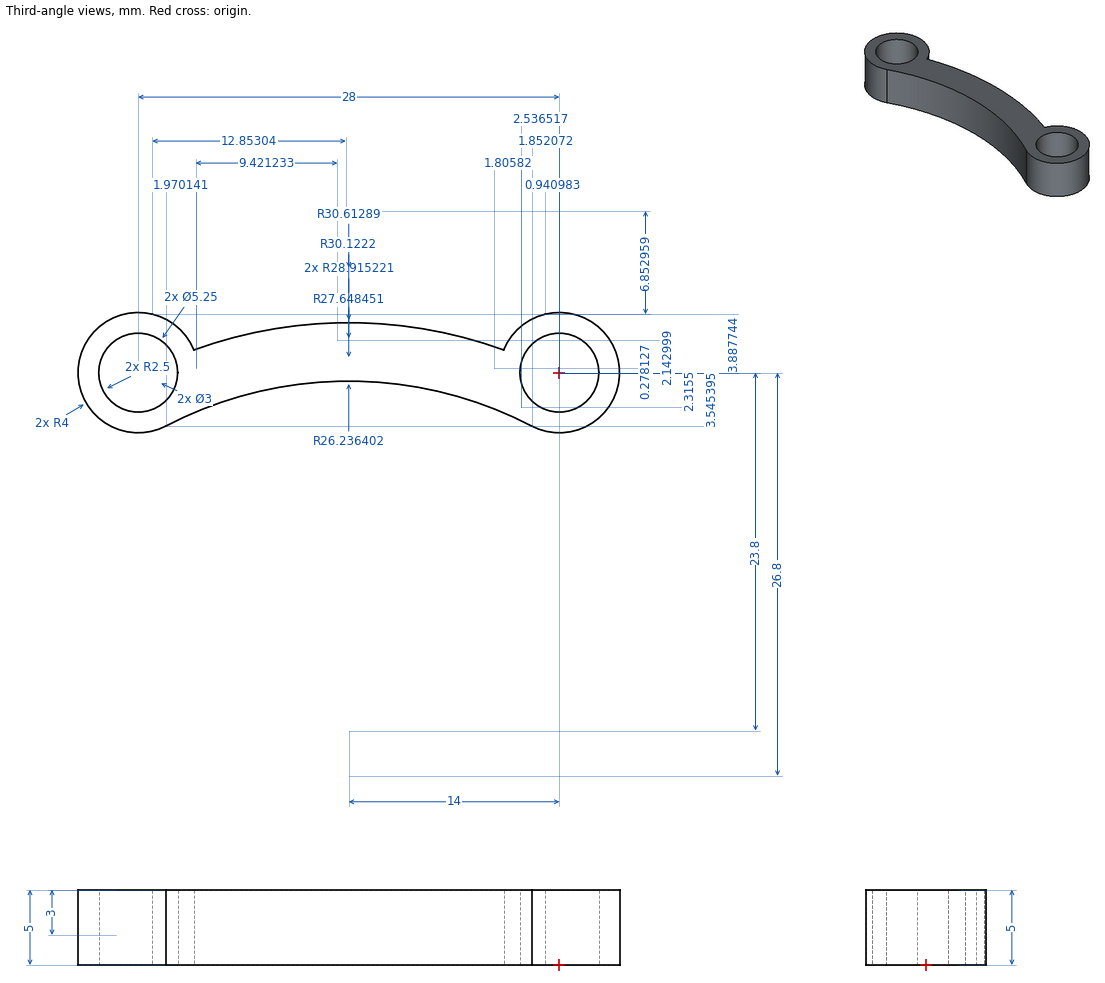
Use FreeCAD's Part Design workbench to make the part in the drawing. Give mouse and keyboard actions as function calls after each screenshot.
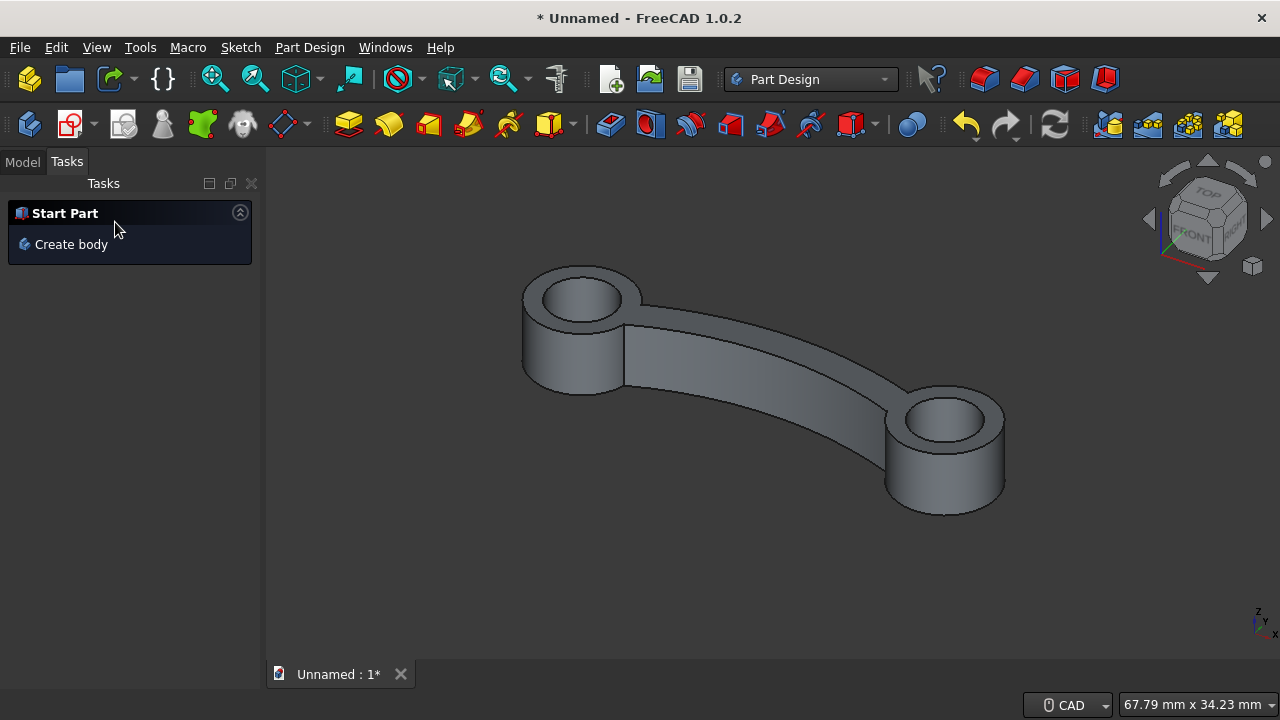
click(897, 403)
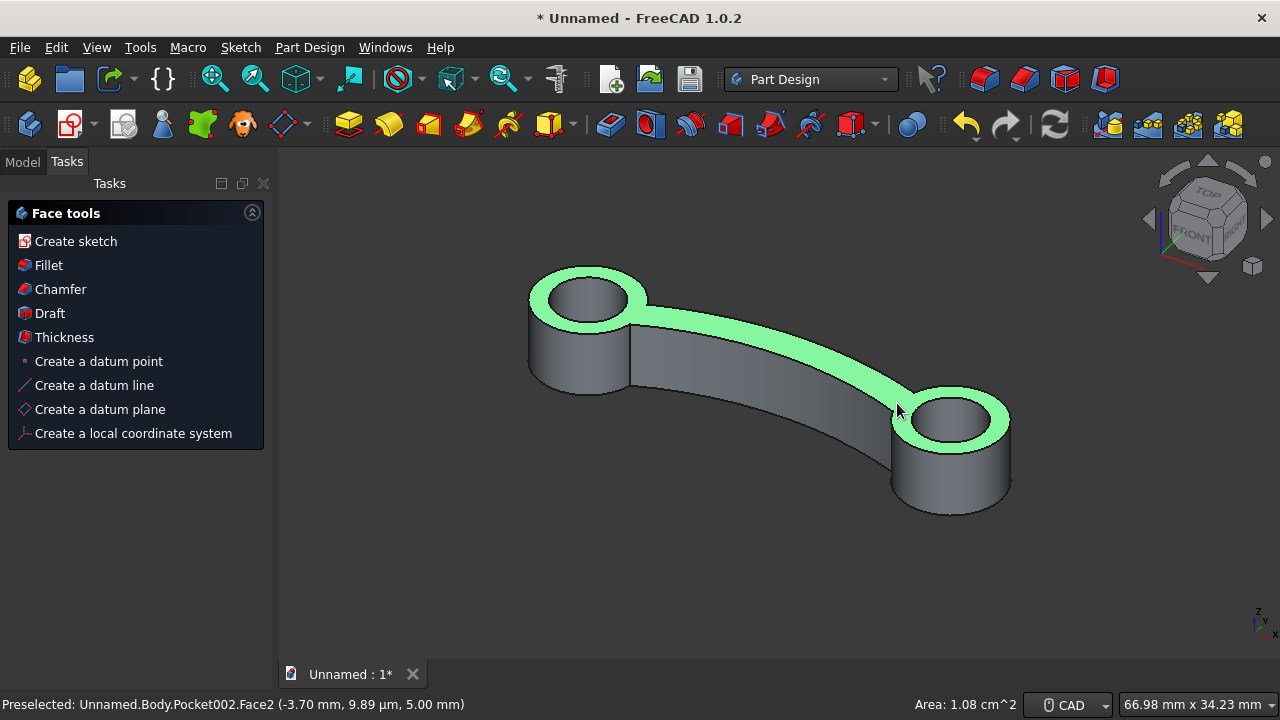
click(70, 124)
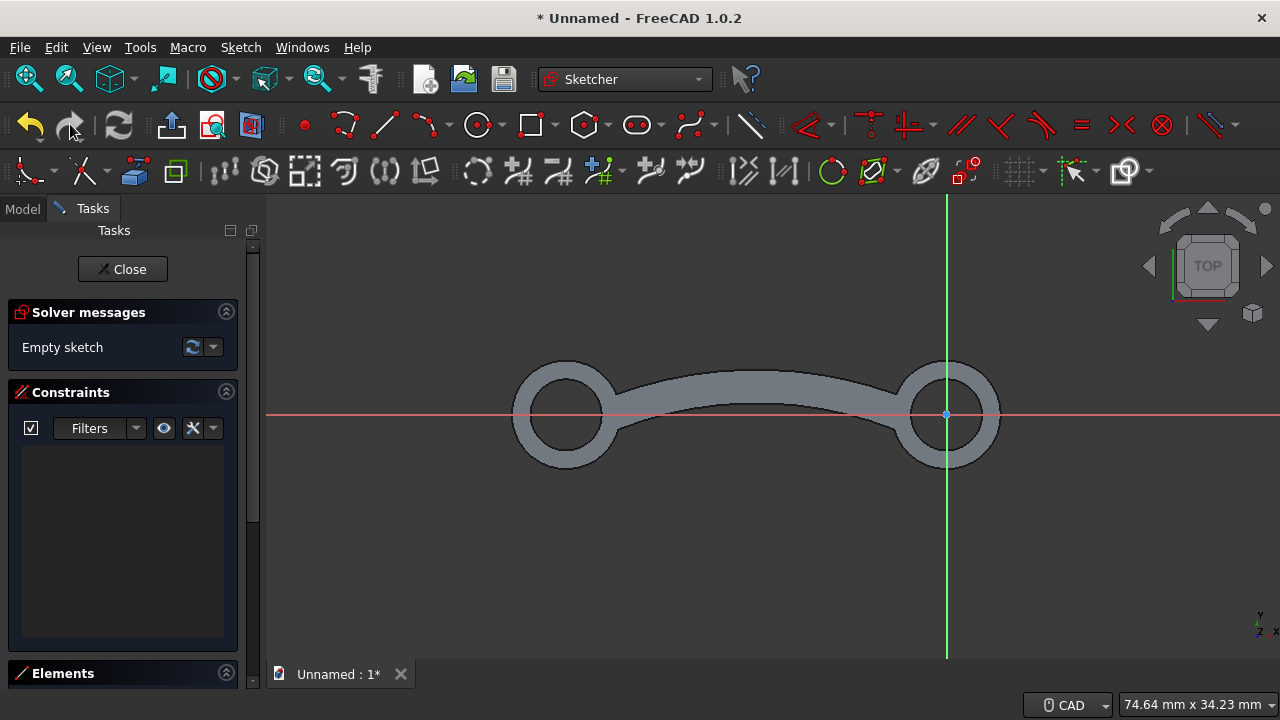
scroll(900, 420, up, 2)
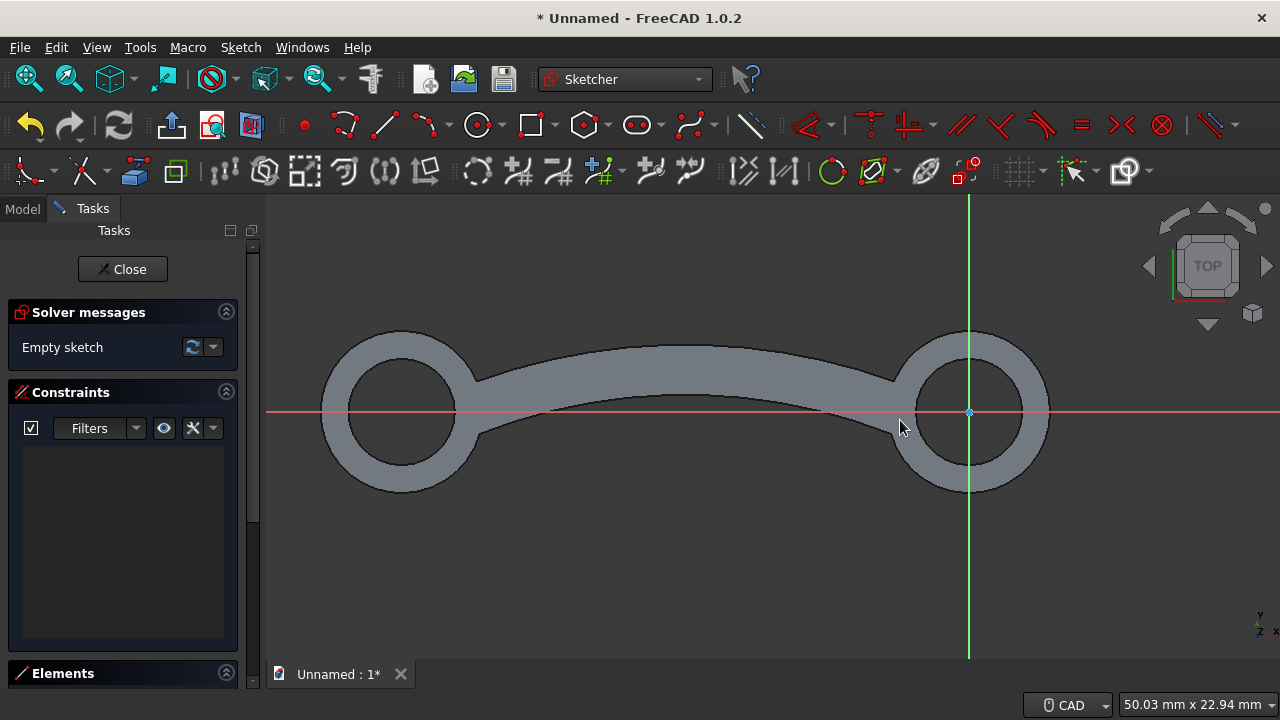
click(346, 126)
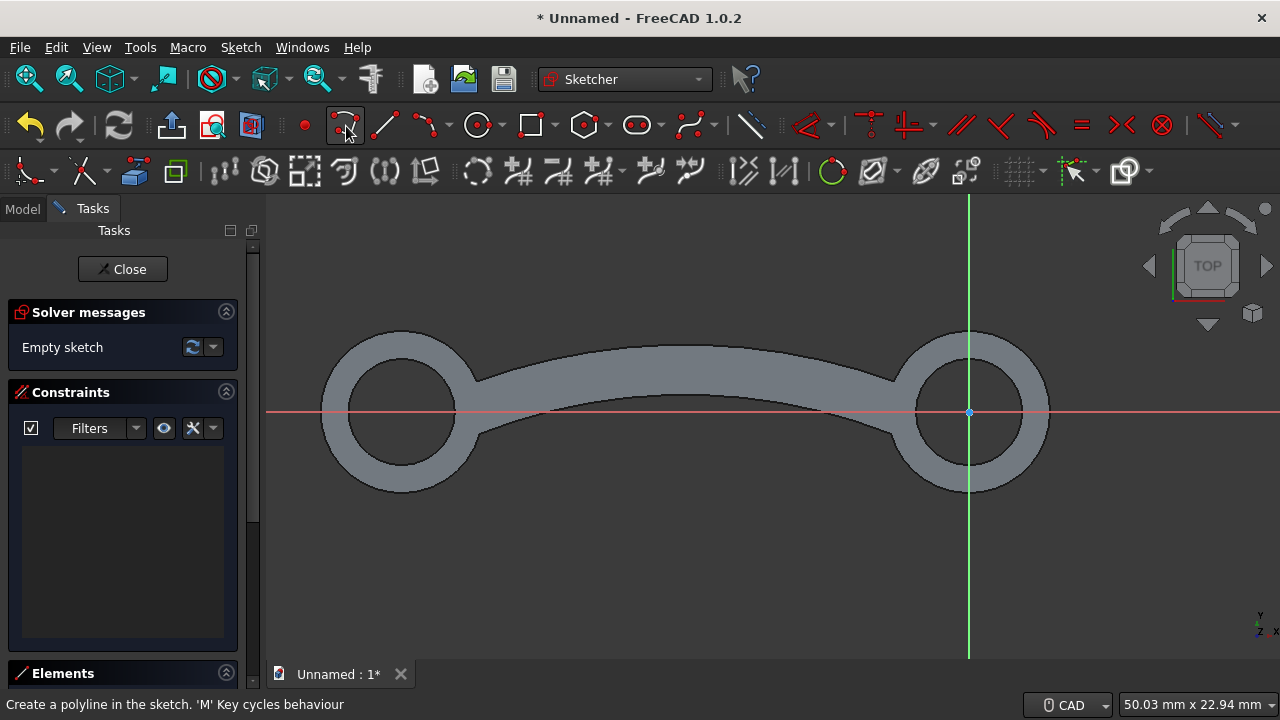
click(932, 484)
click(918, 459)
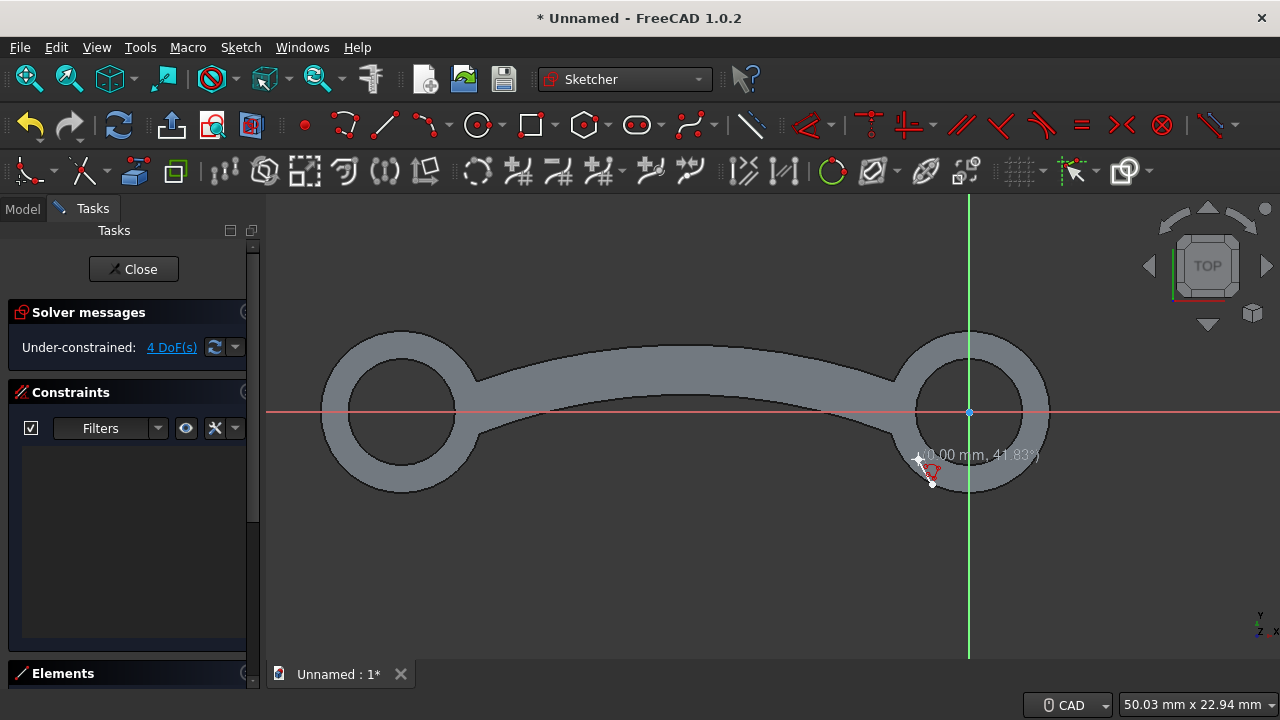
scroll(881, 406, up, 6)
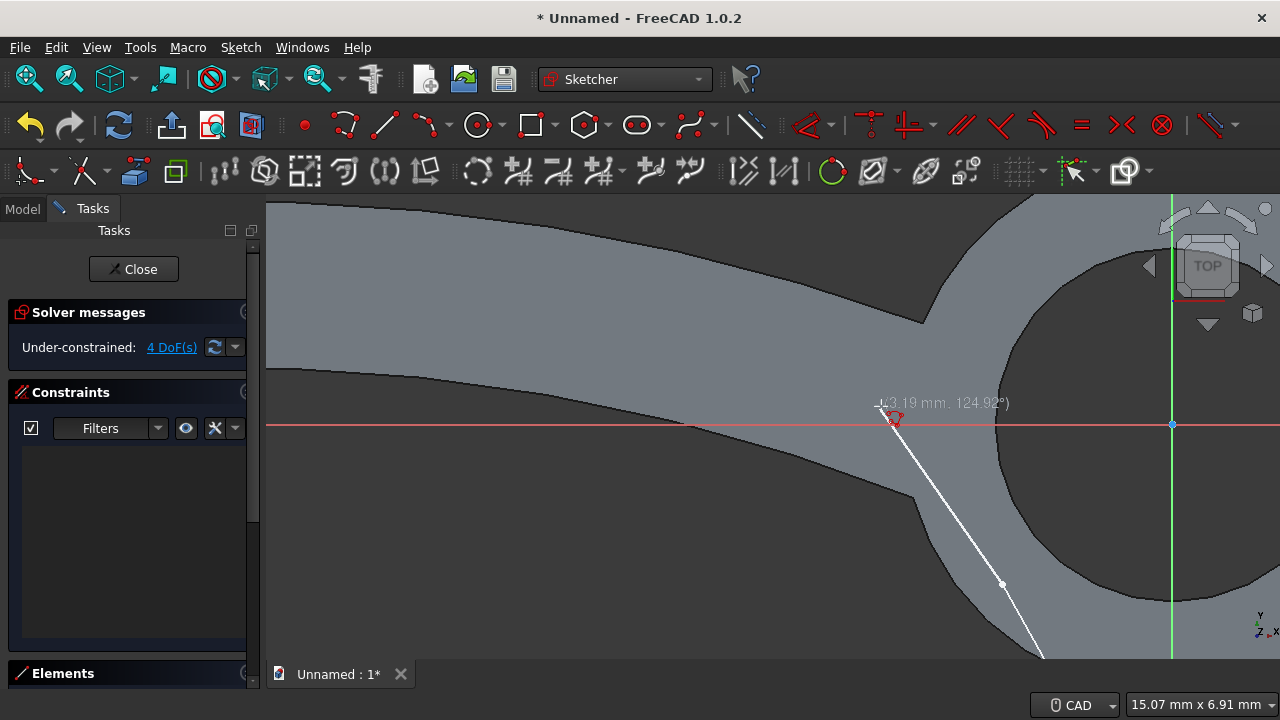
click(880, 406)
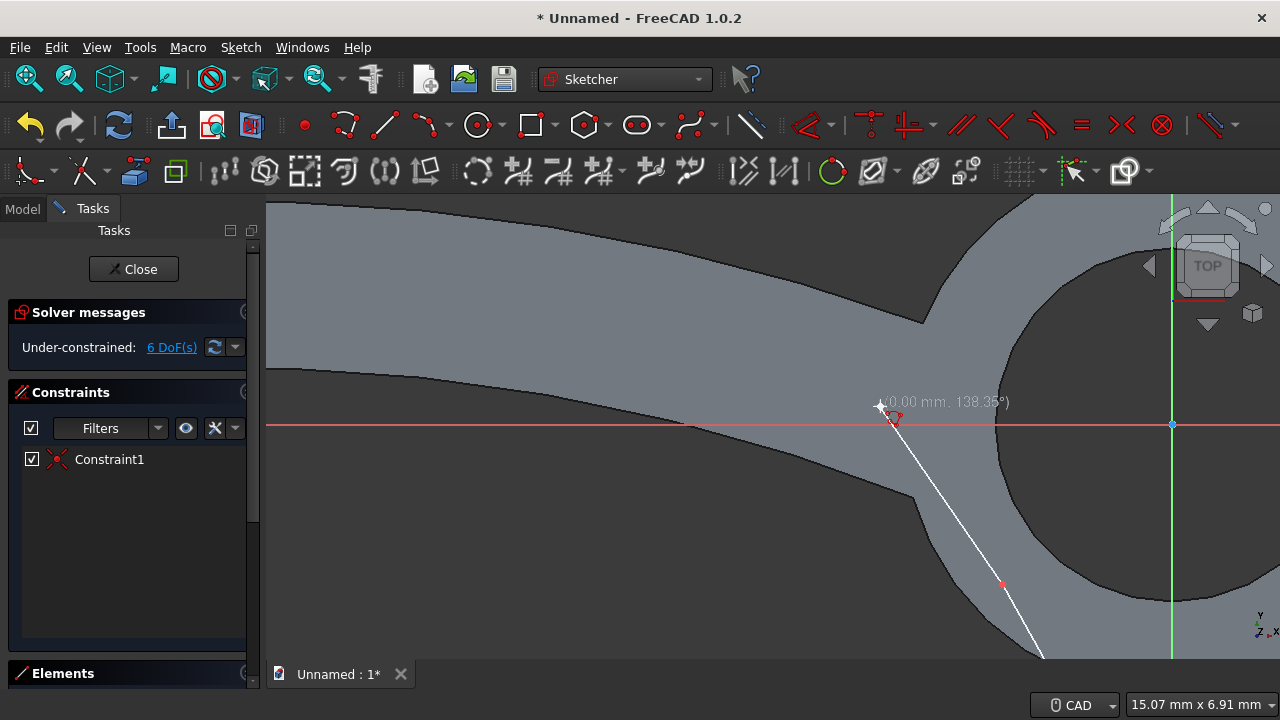
scroll(882, 407, down, 6)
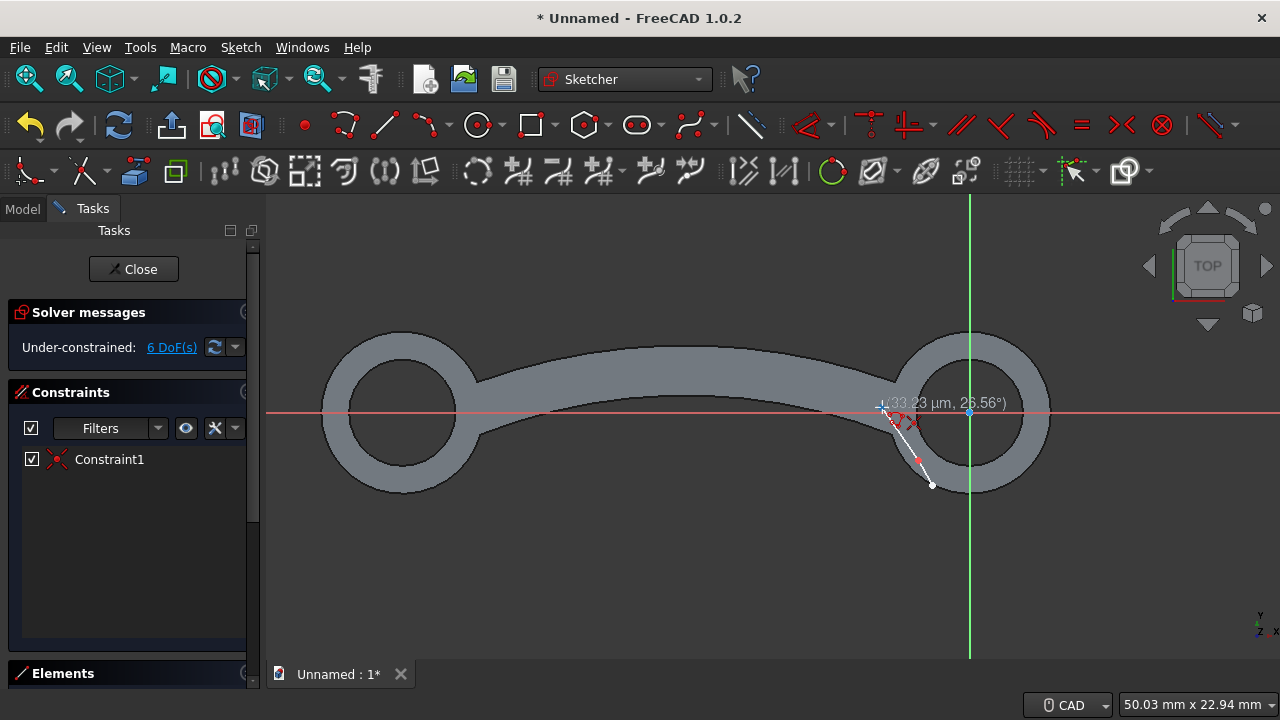
click(671, 369)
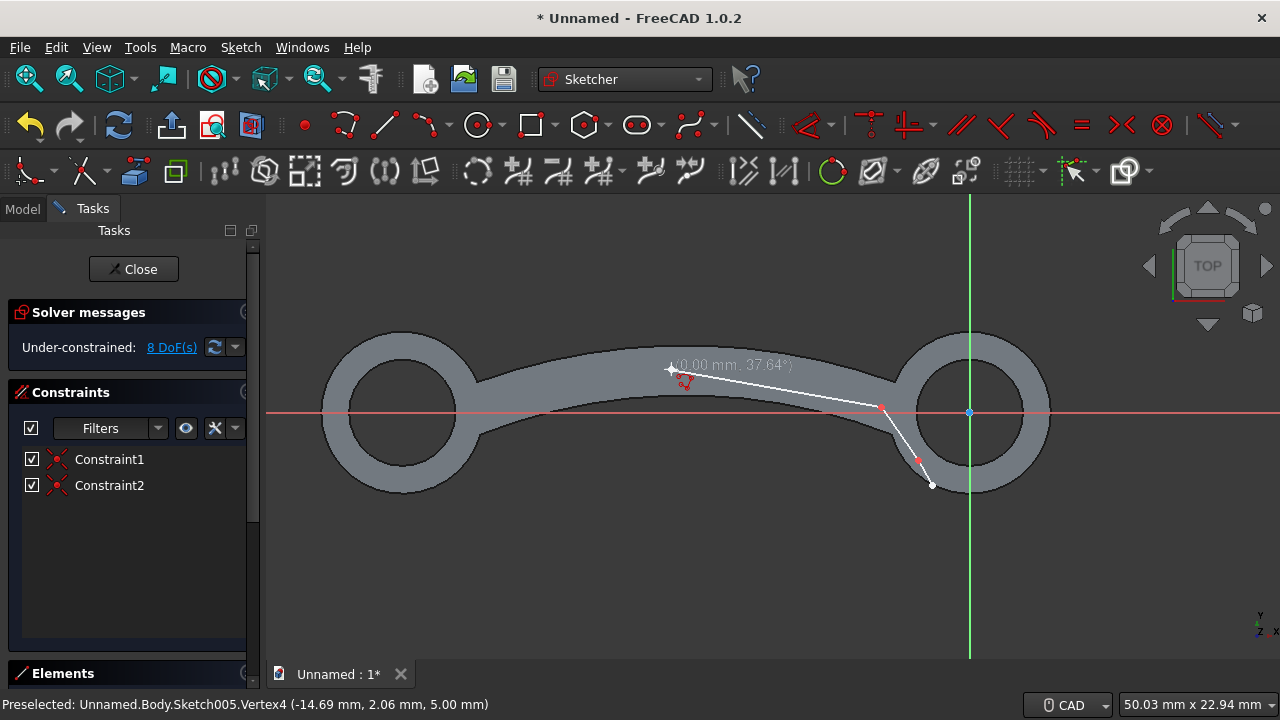
scroll(480, 407, up, 6)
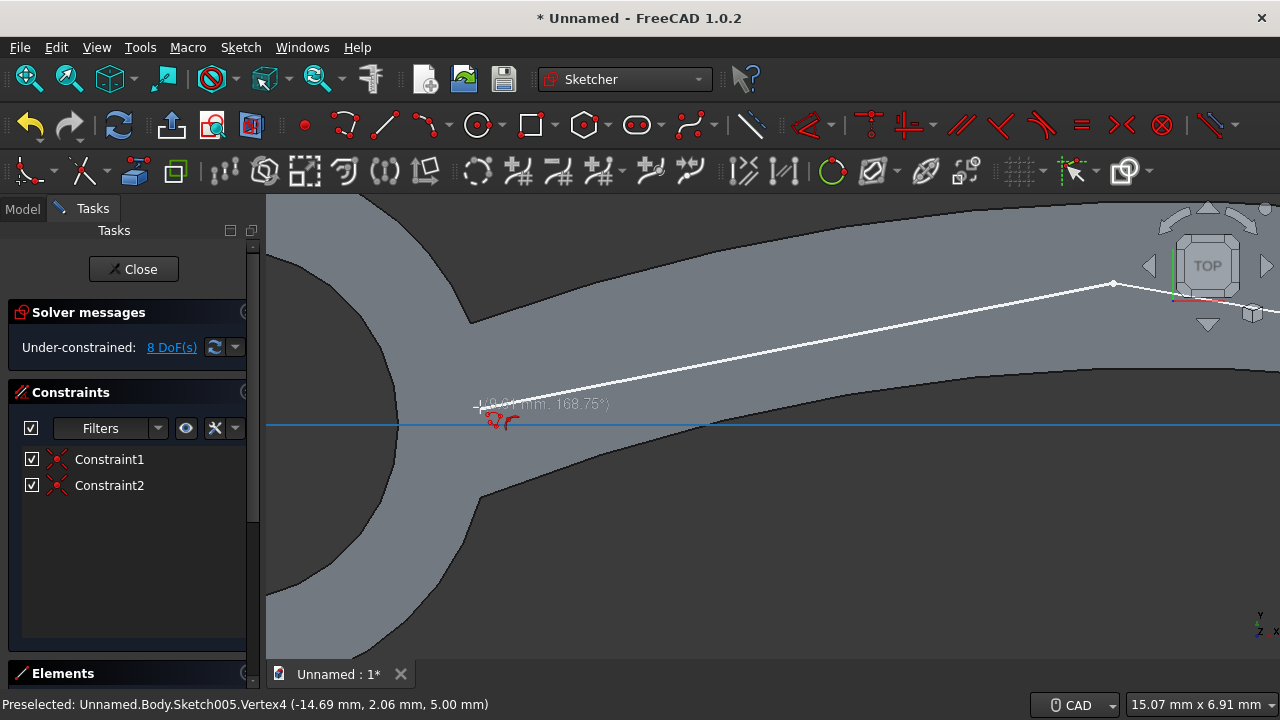
click(479, 406)